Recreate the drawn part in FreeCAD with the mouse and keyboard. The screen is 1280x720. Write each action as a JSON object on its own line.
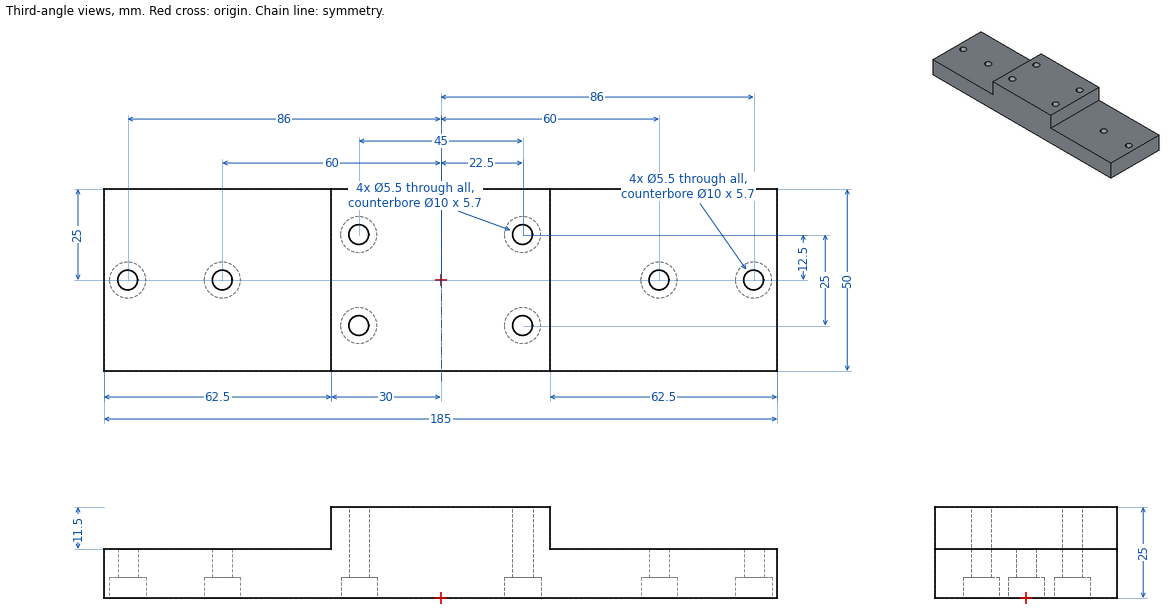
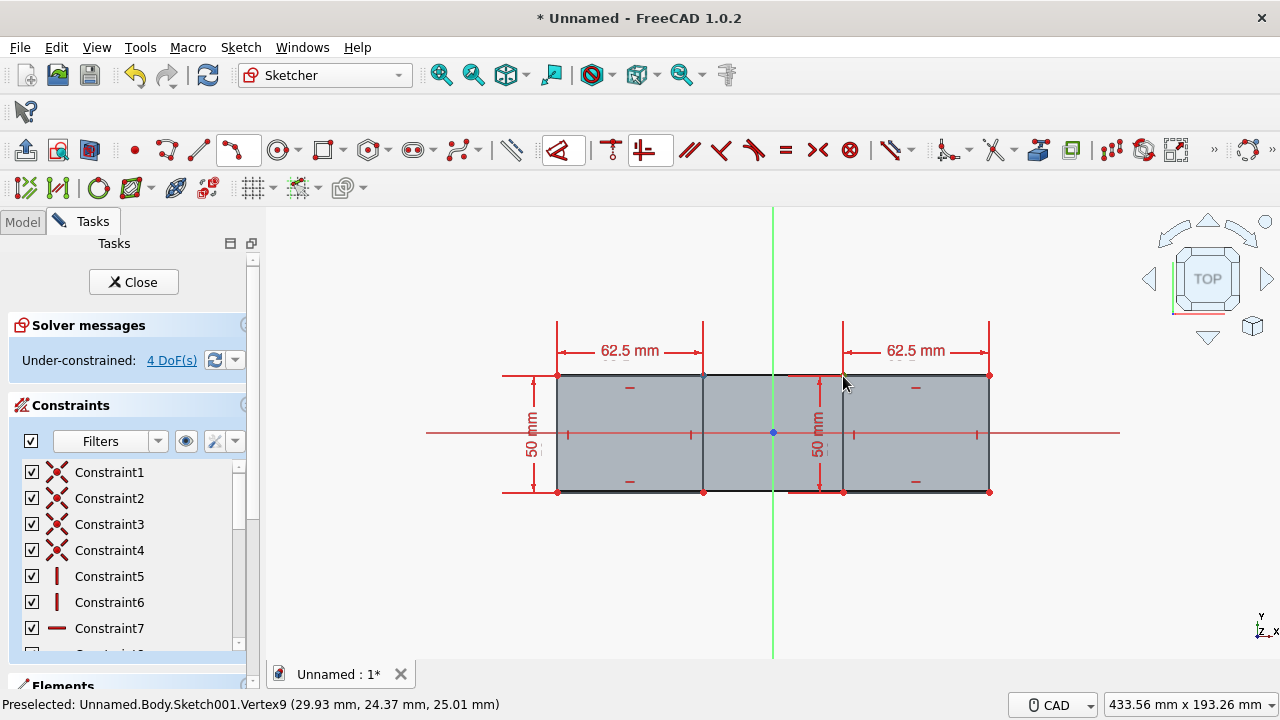
{"action": "left_click", "coordinate": [773, 603]}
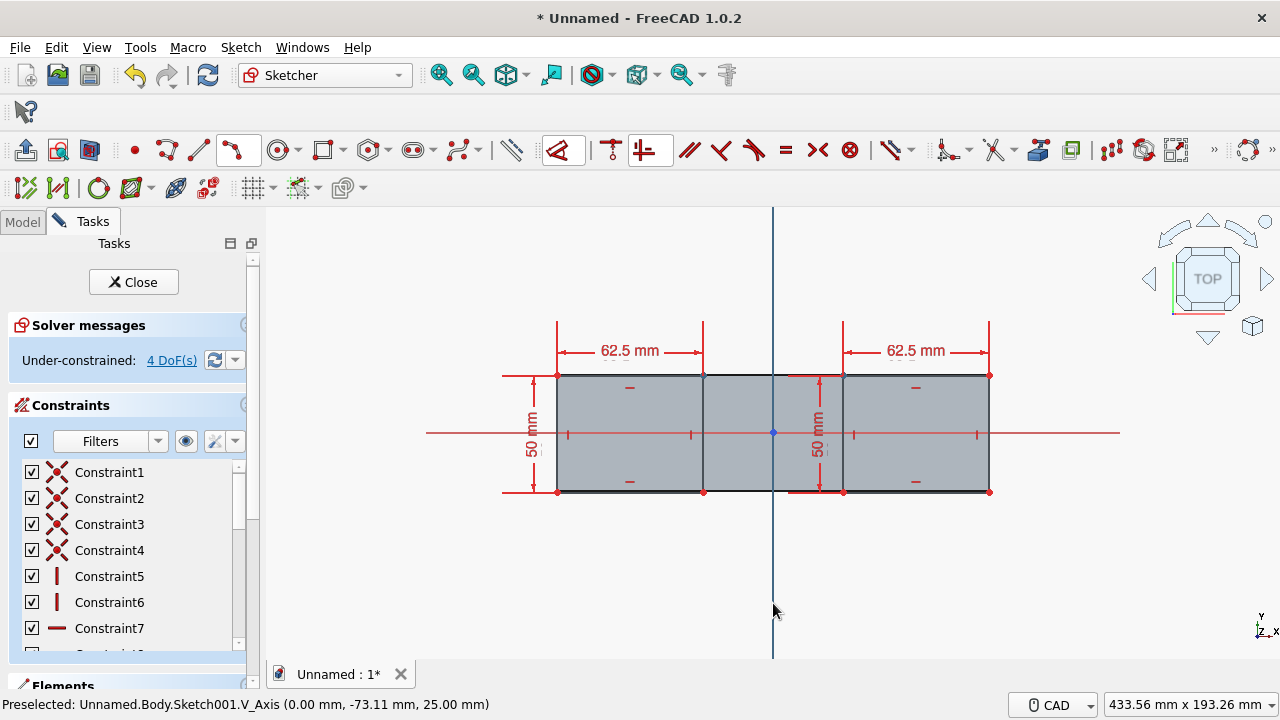
{"action": "left_click", "coordinate": [818, 150]}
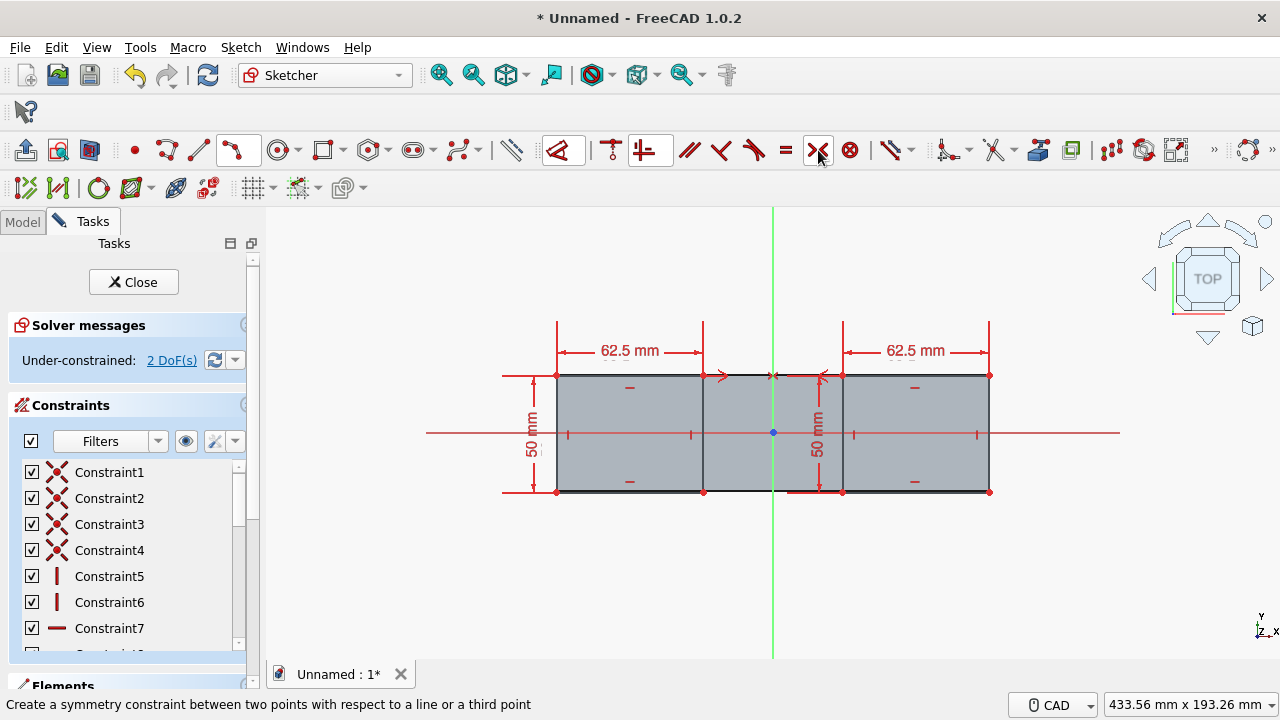
{"action": "key", "text": "d"}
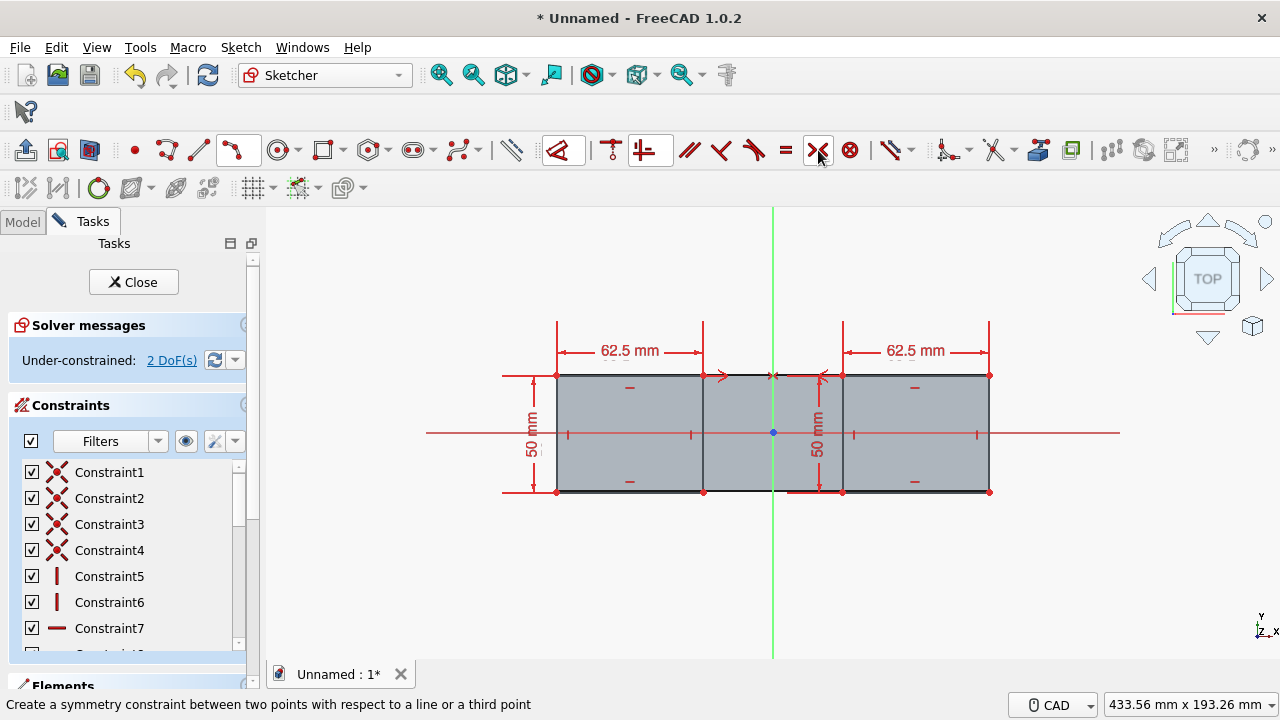
{"action": "left_click", "coordinate": [557, 376]}
{"action": "left_click", "coordinate": [523, 404]}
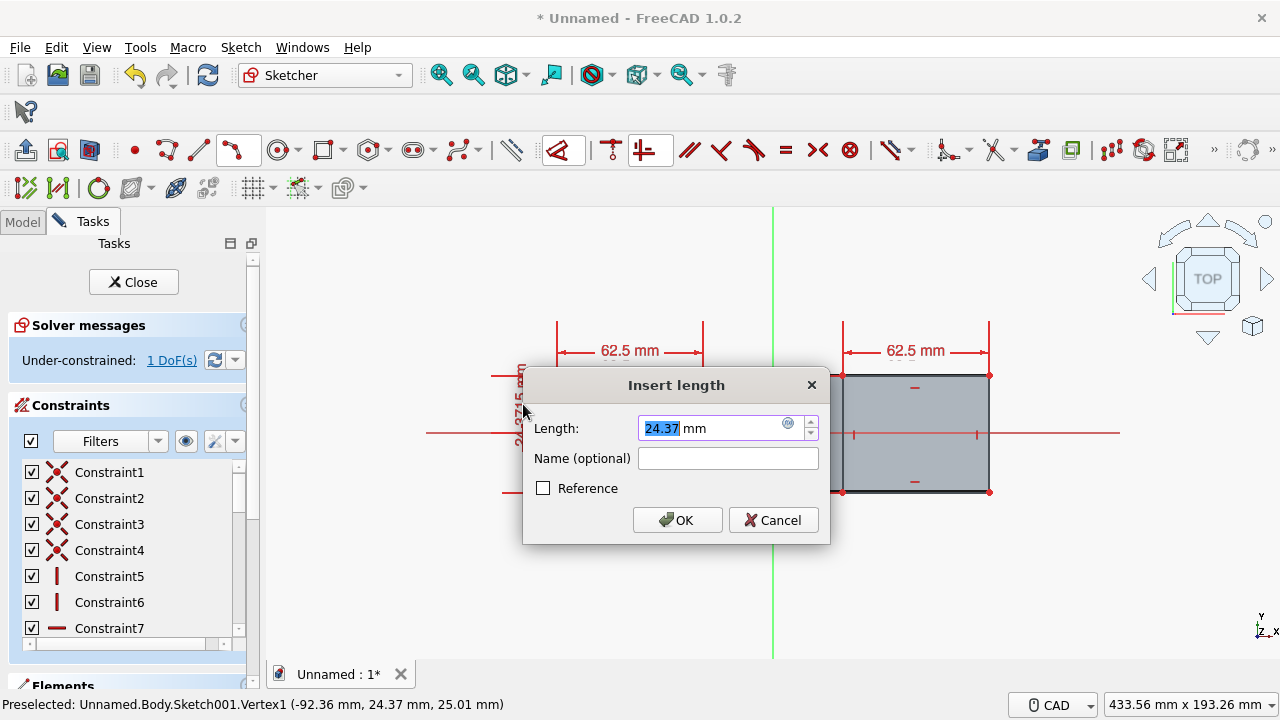
{"action": "type", "text": "25"}
{"action": "key", "text": "Return"}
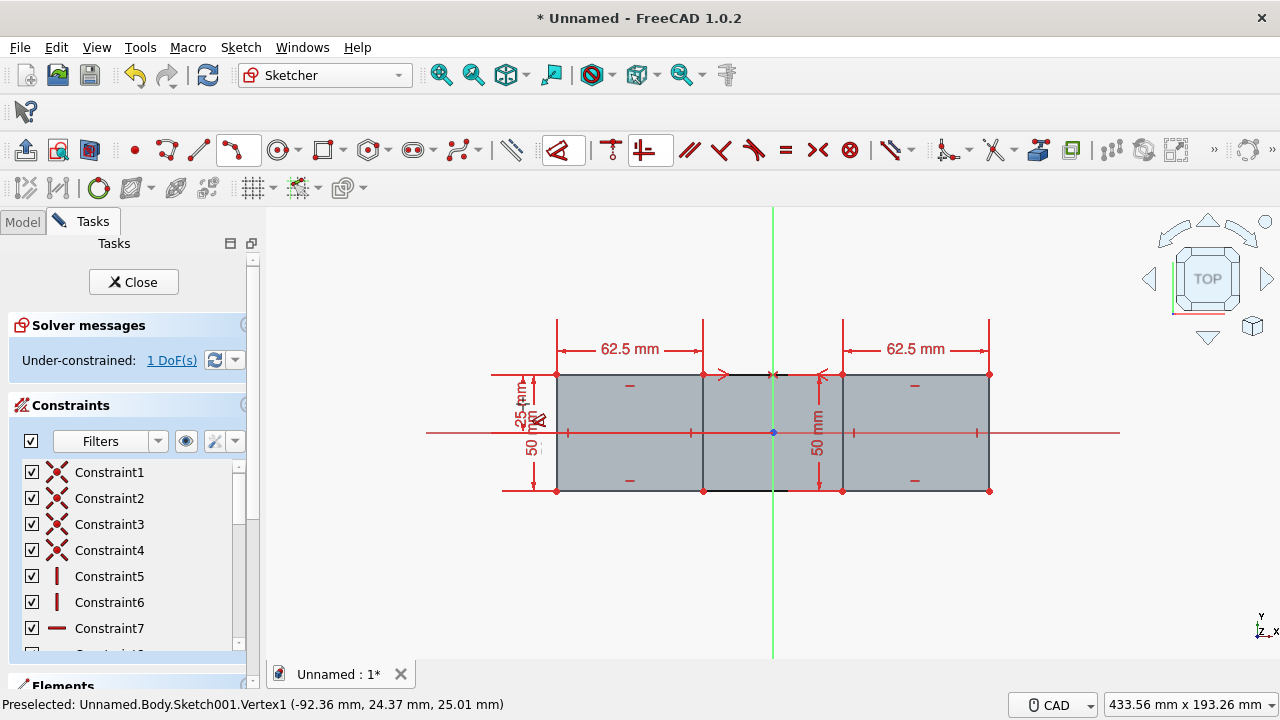
{"action": "left_click", "coordinate": [703, 491]}
{"action": "left_click", "coordinate": [738, 525]}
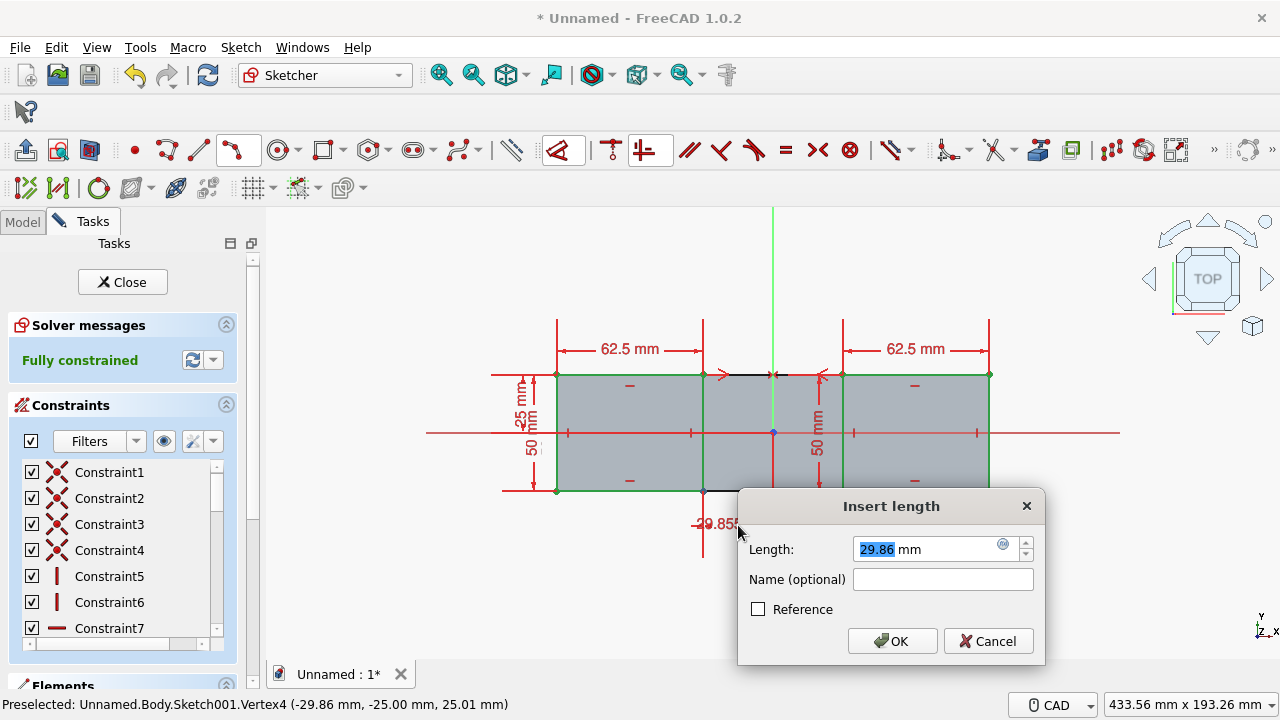
{"action": "type", "text": "30"}
{"action": "key", "text": "Return"}
{"action": "key", "text": "Escape"}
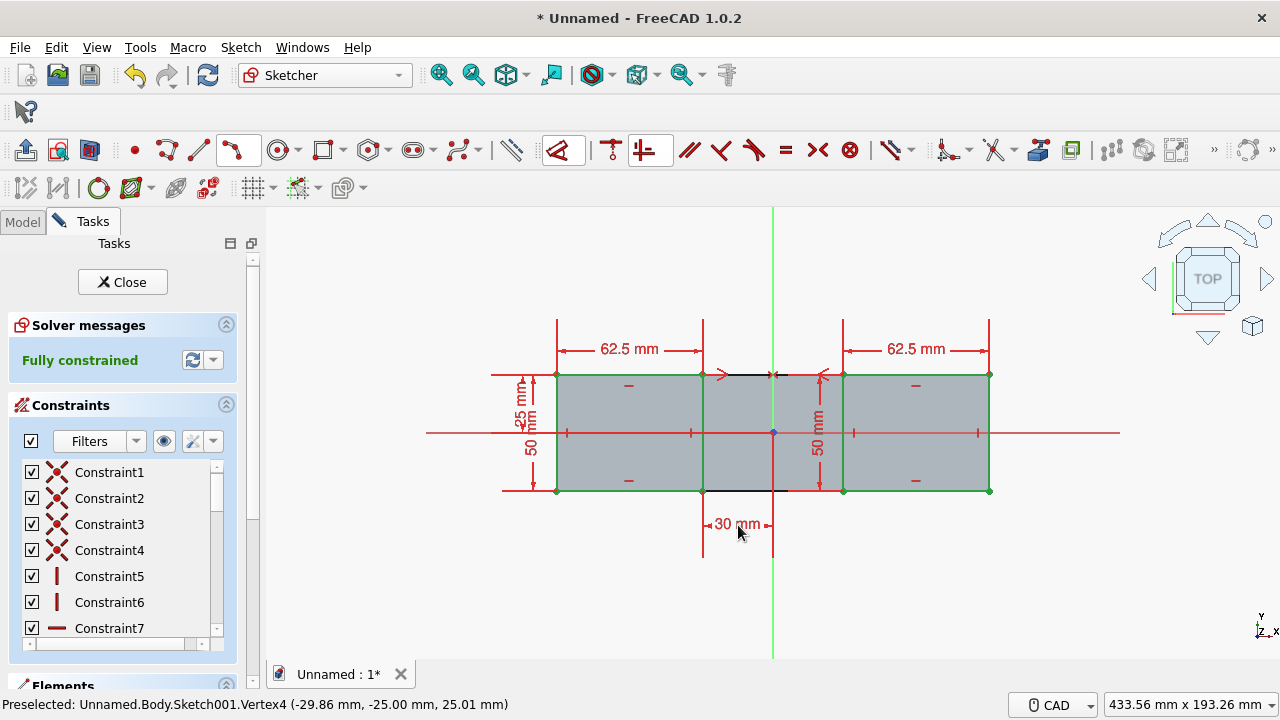
{"action": "left_click", "coordinate": [123, 282]}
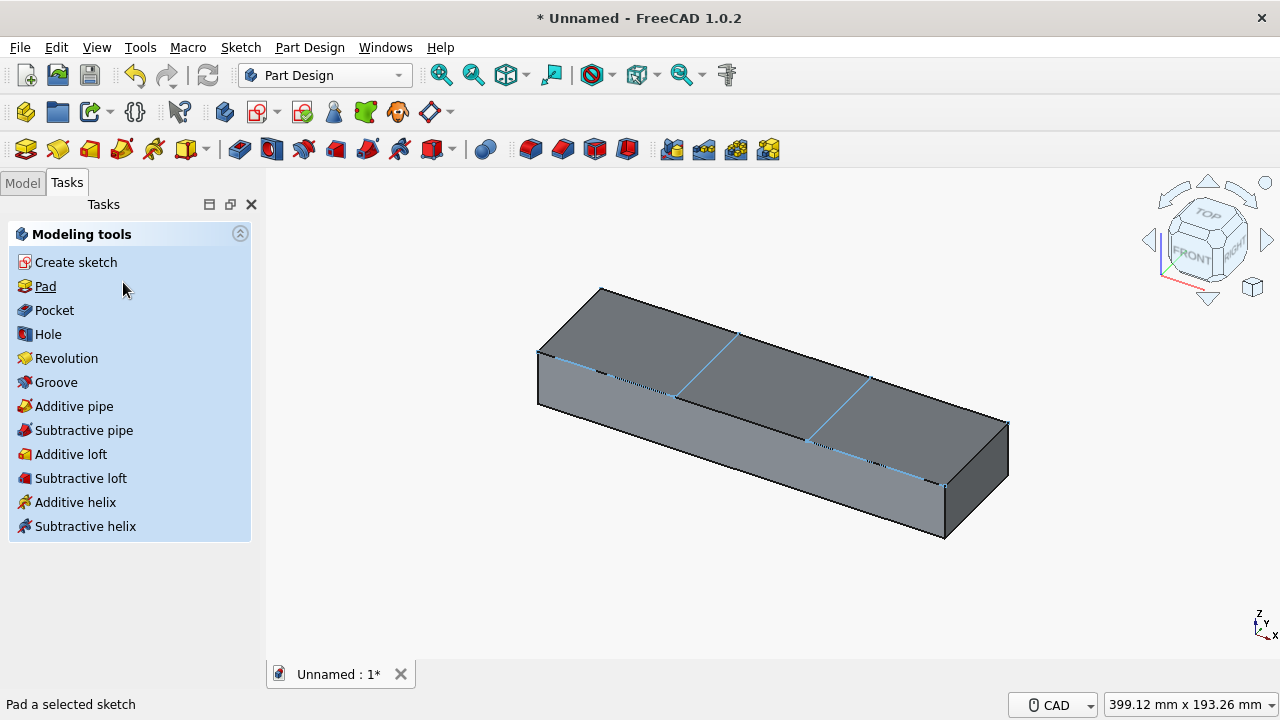
{"action": "left_click", "coordinate": [240, 150]}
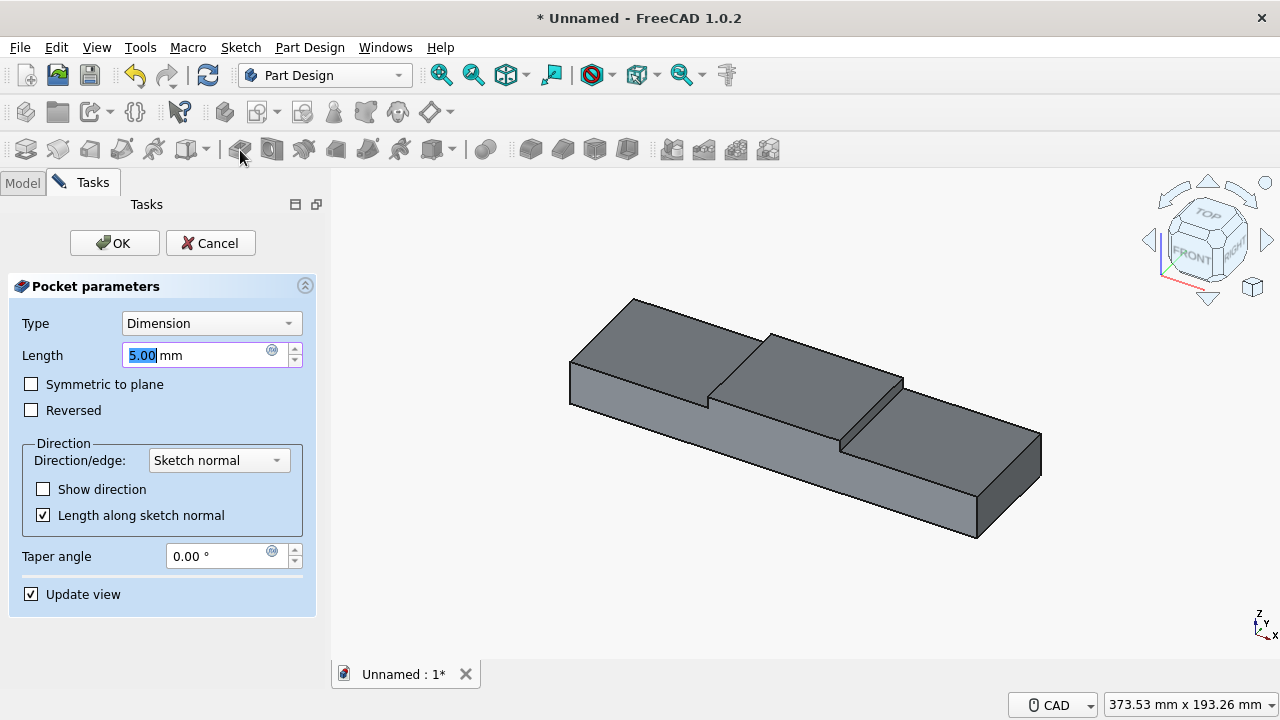
{"action": "type", "text": "11.5"}
{"action": "key", "text": "Tab"}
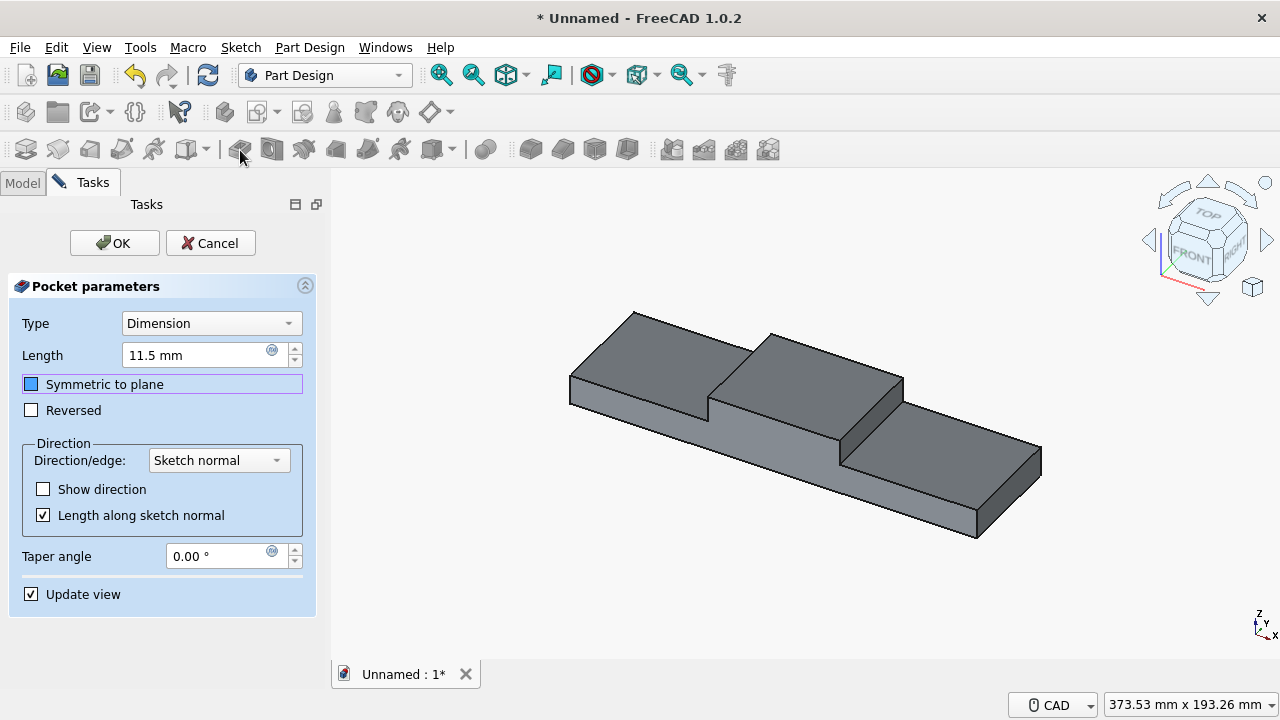
{"action": "left_click", "coordinate": [115, 243]}